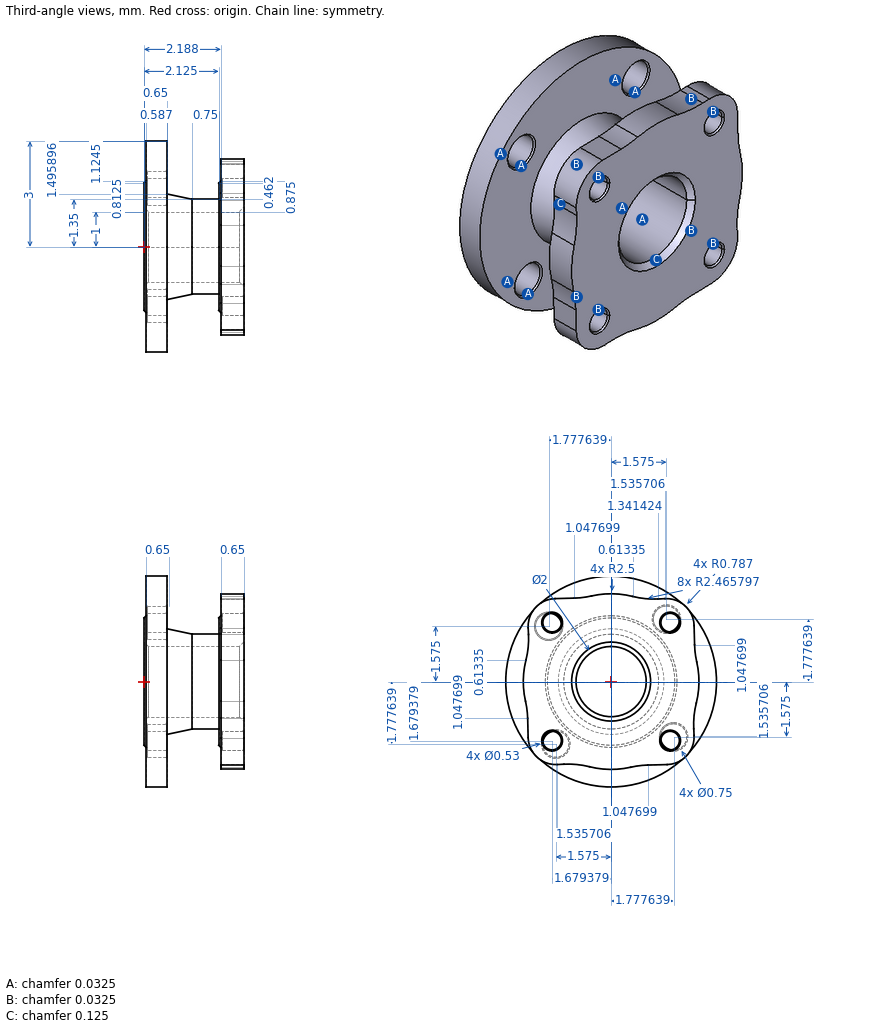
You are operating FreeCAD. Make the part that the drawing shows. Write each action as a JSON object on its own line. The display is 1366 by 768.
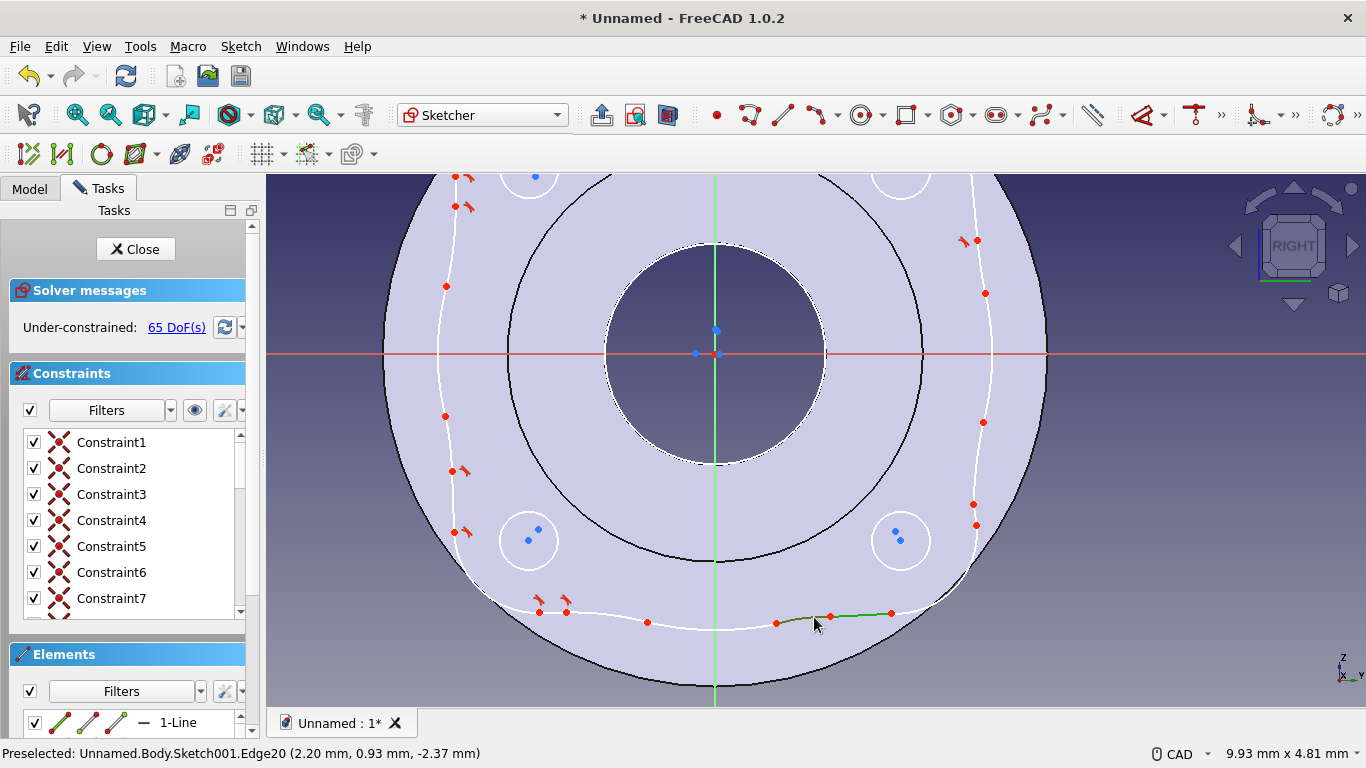
{"action": "key", "text": "t"}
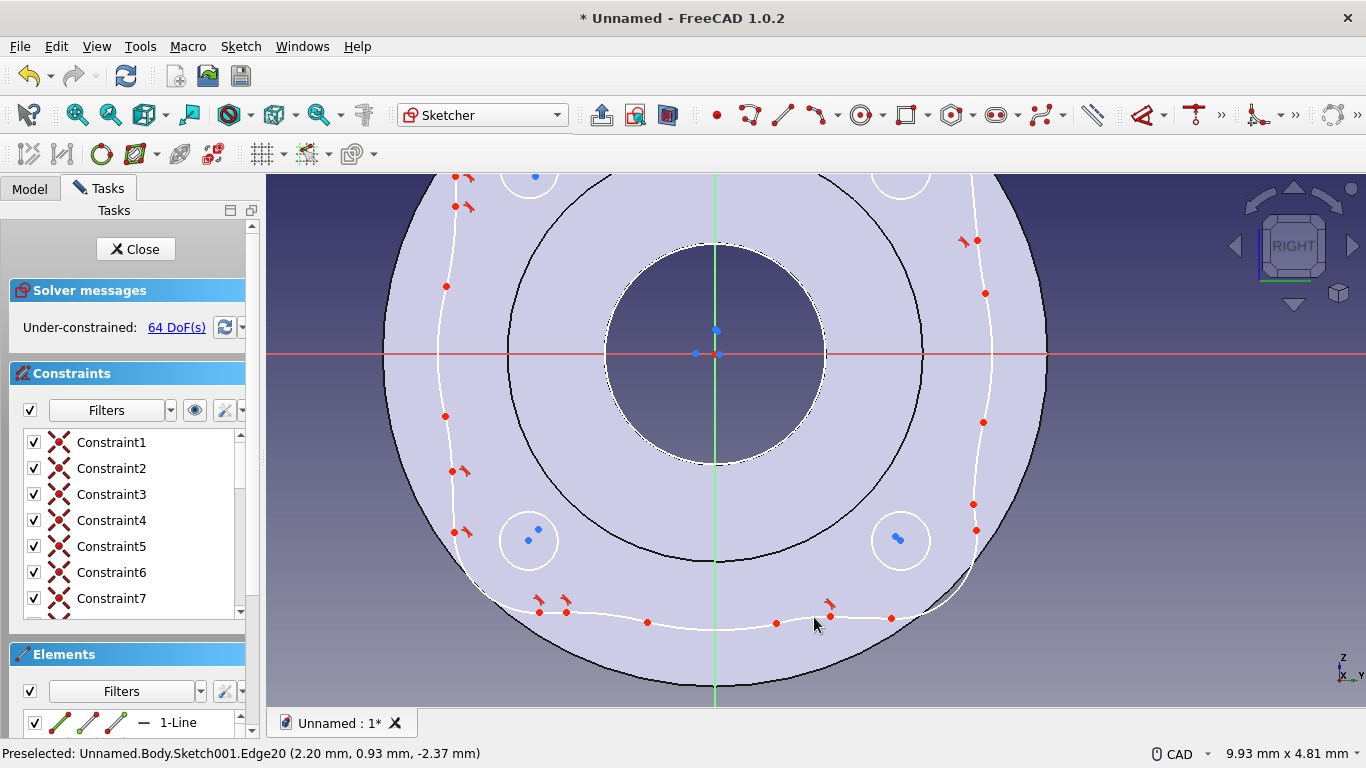
{"action": "left_click", "coordinate": [849, 618]}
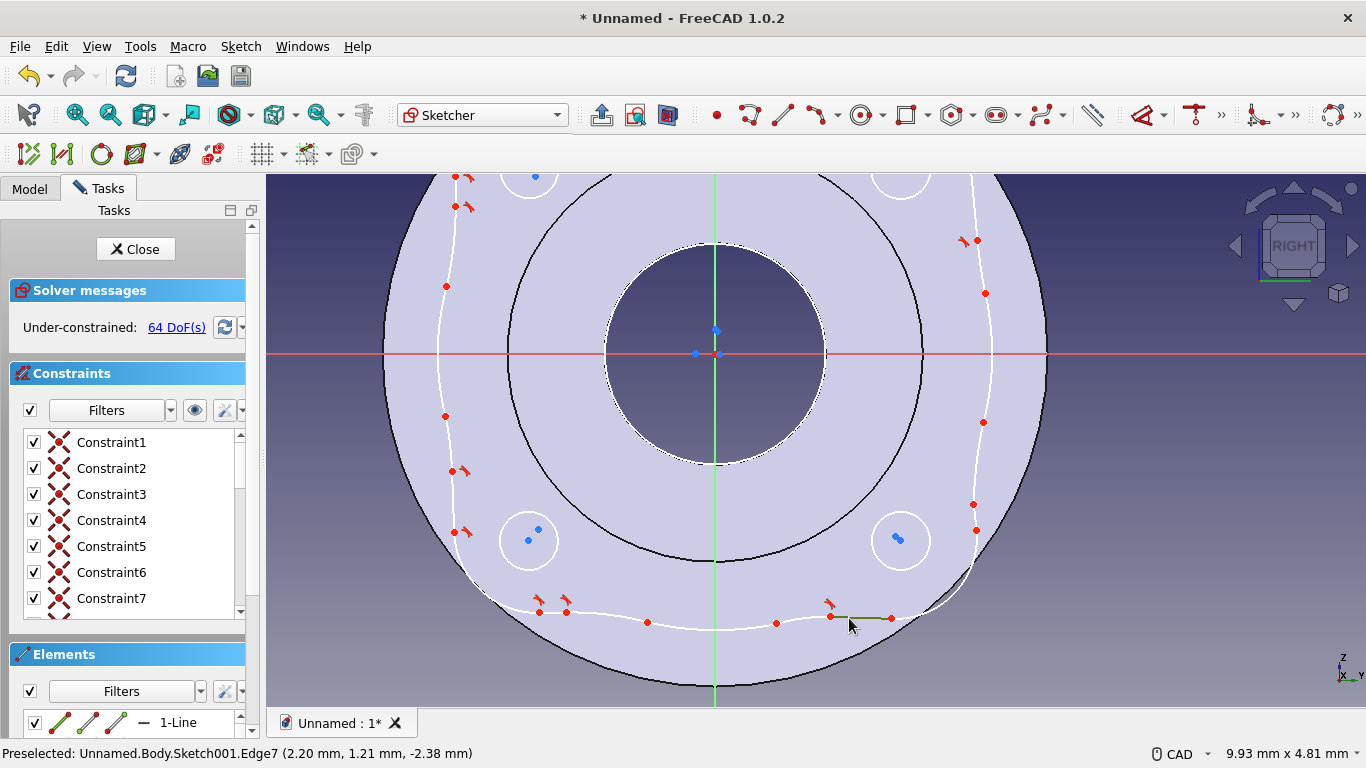
{"action": "left_click", "coordinate": [932, 610]}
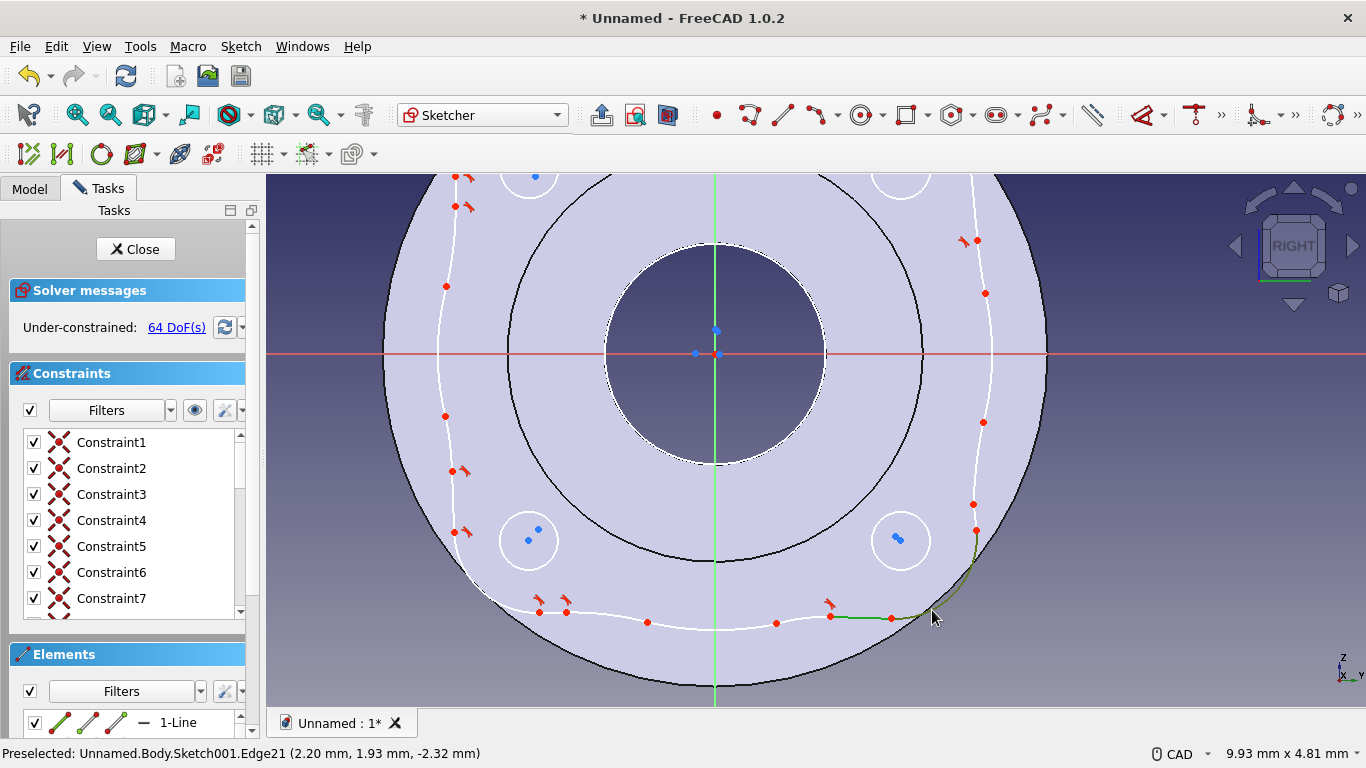
{"action": "key", "text": "t"}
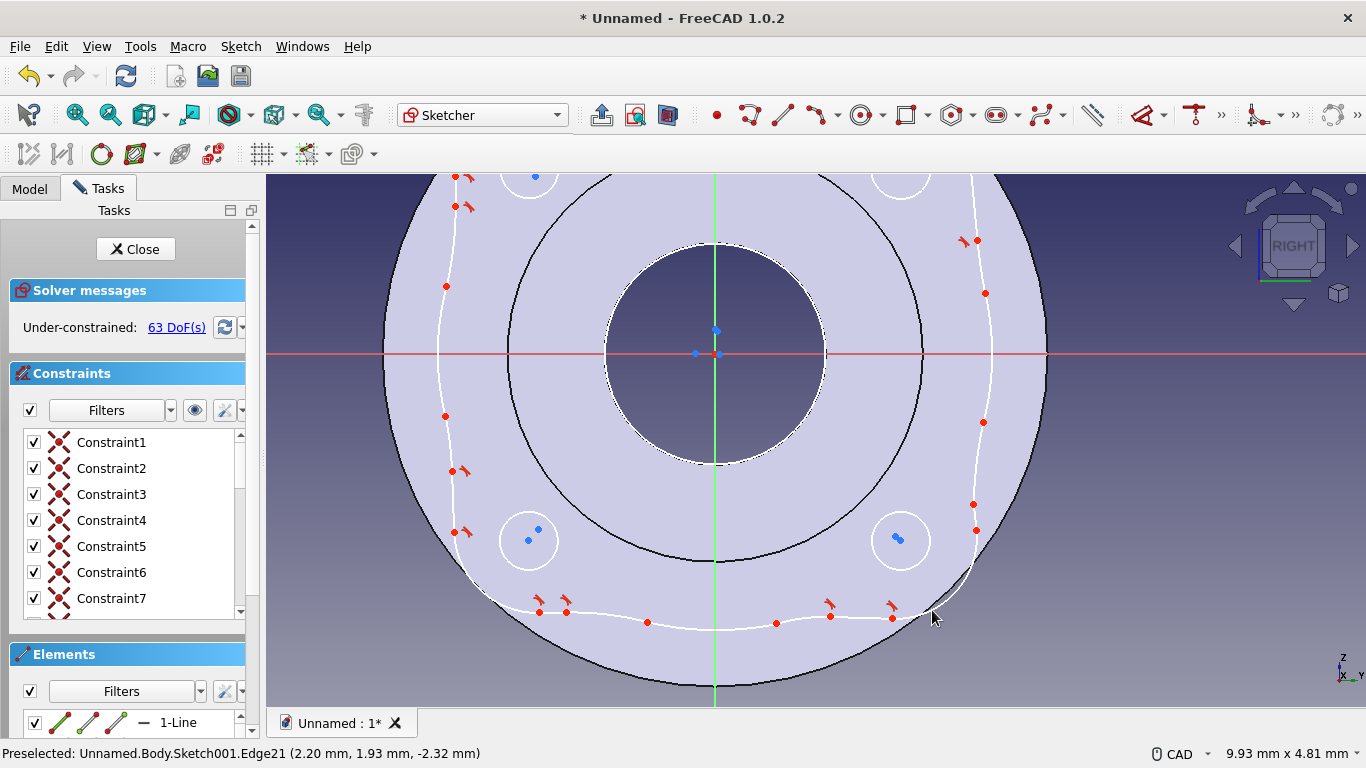
{"action": "scroll", "coordinate": [976, 520], "scroll_direction": "up", "scroll_amount": 2}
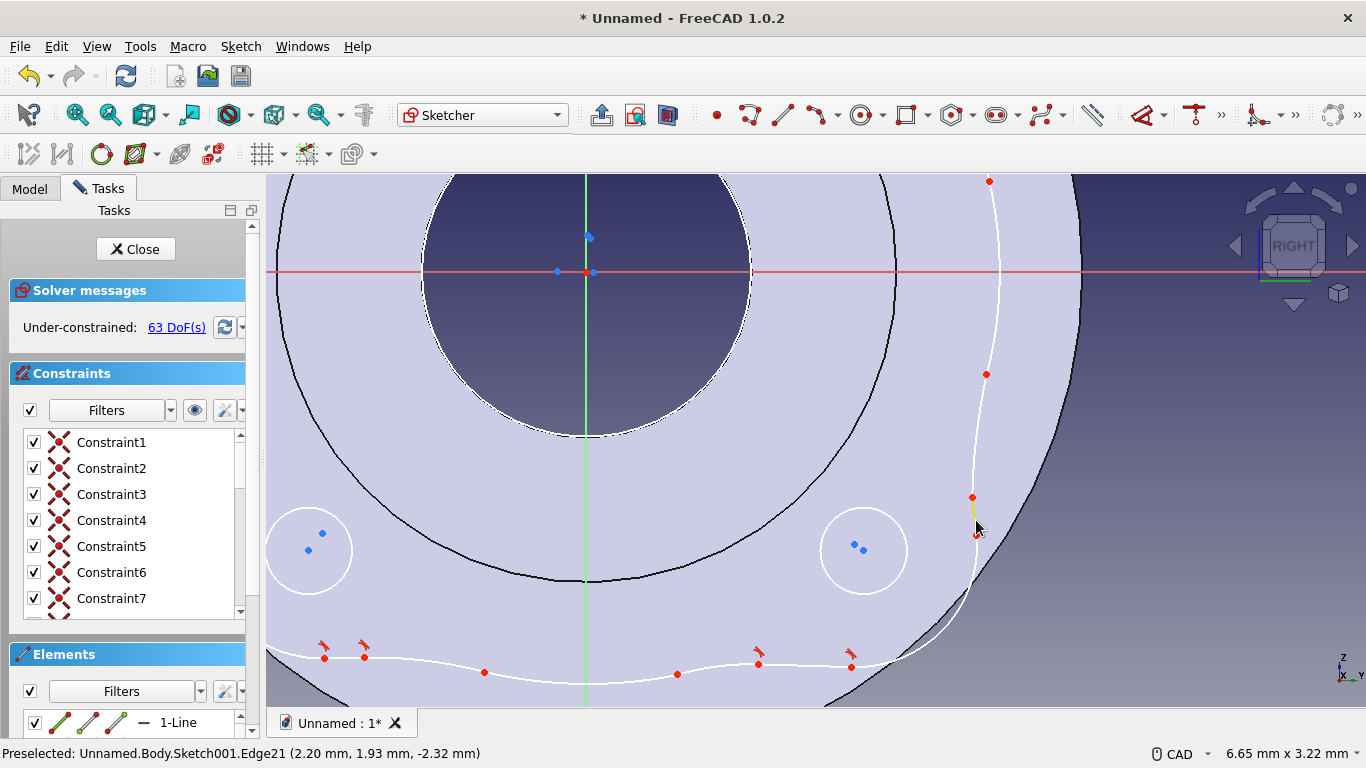
{"action": "left_click", "coordinate": [975, 520]}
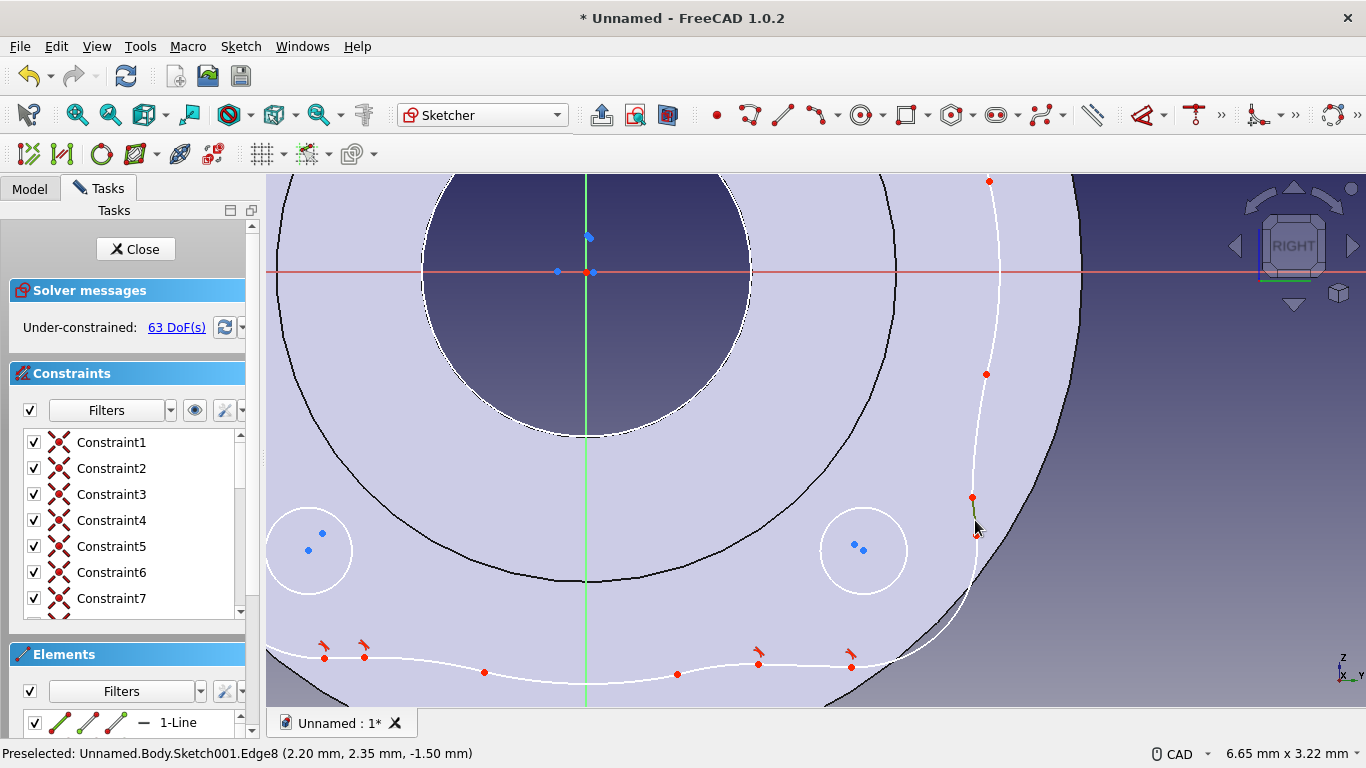
{"action": "left_click", "coordinate": [911, 654]}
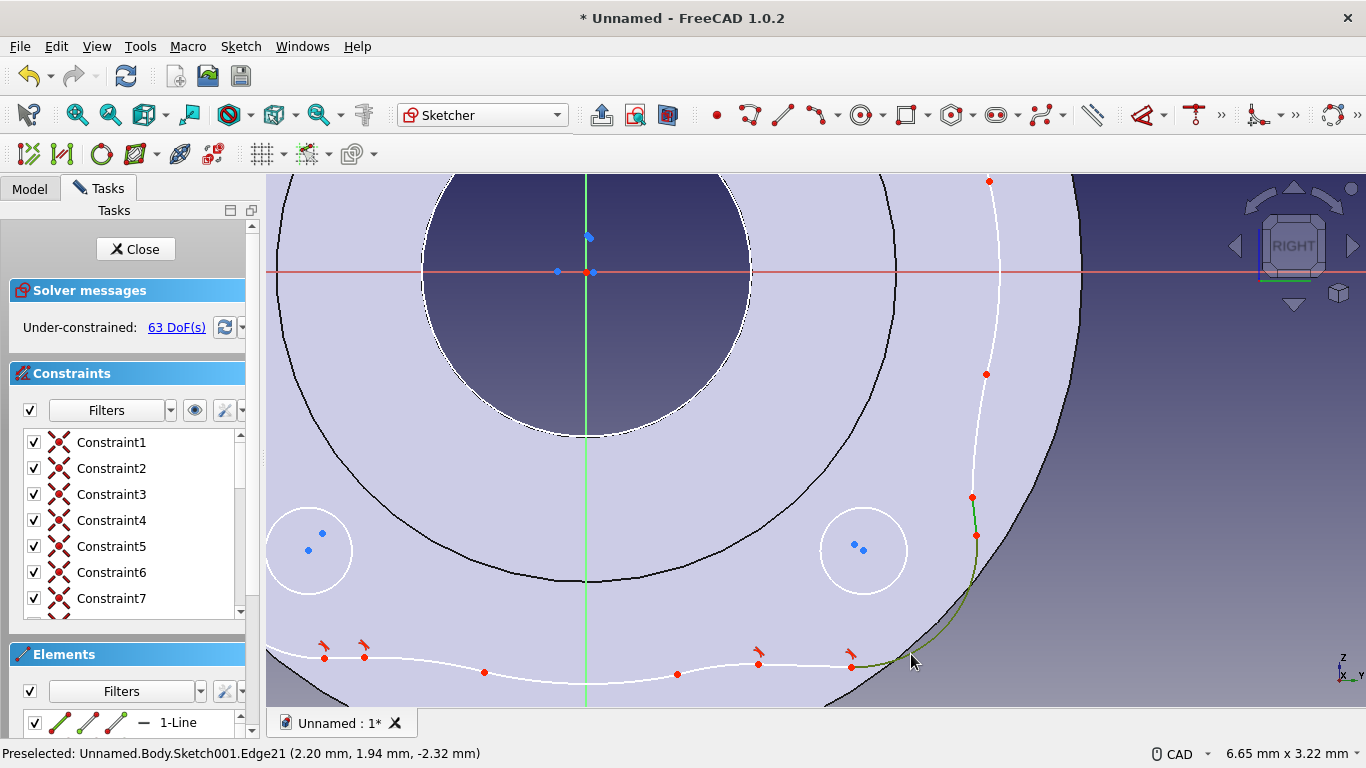
{"action": "key", "text": "t"}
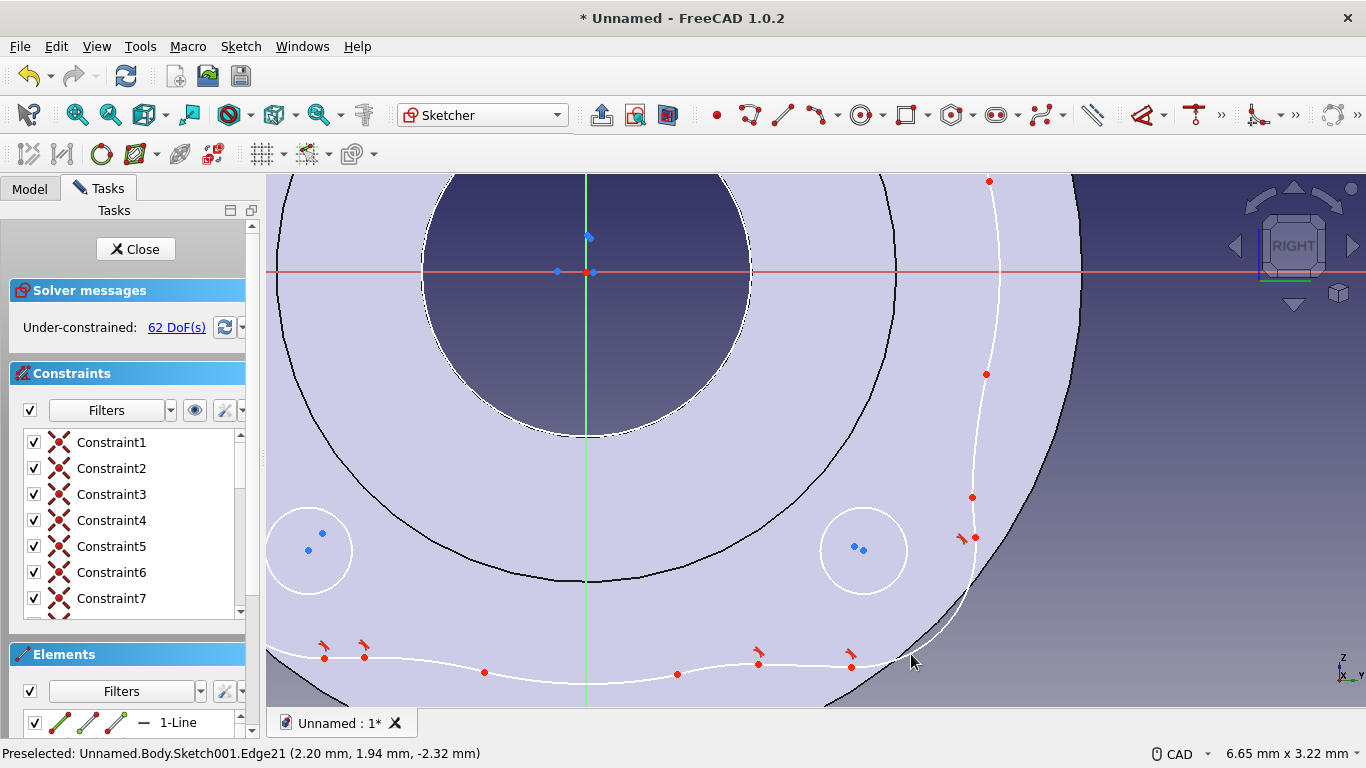
{"action": "left_click", "coordinate": [974, 525]}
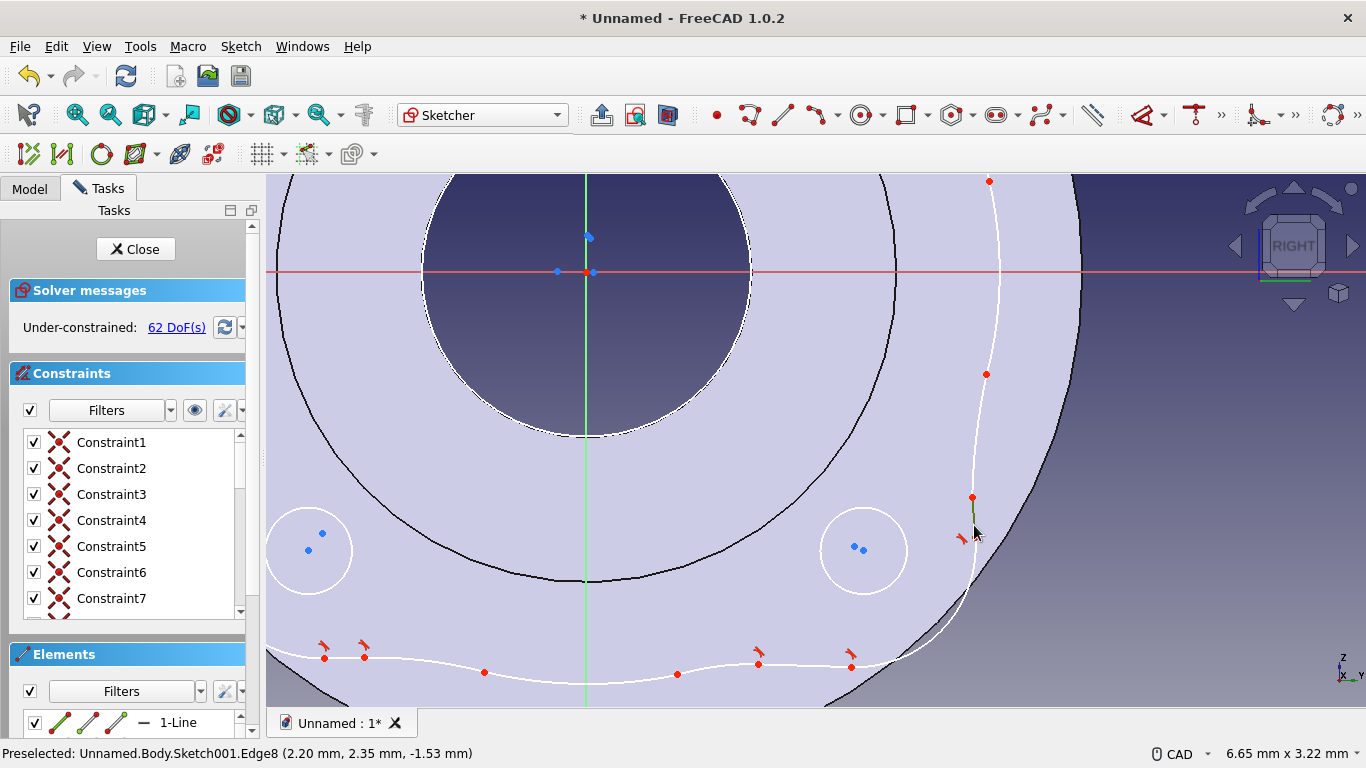
{"action": "left_click", "coordinate": [980, 411]}